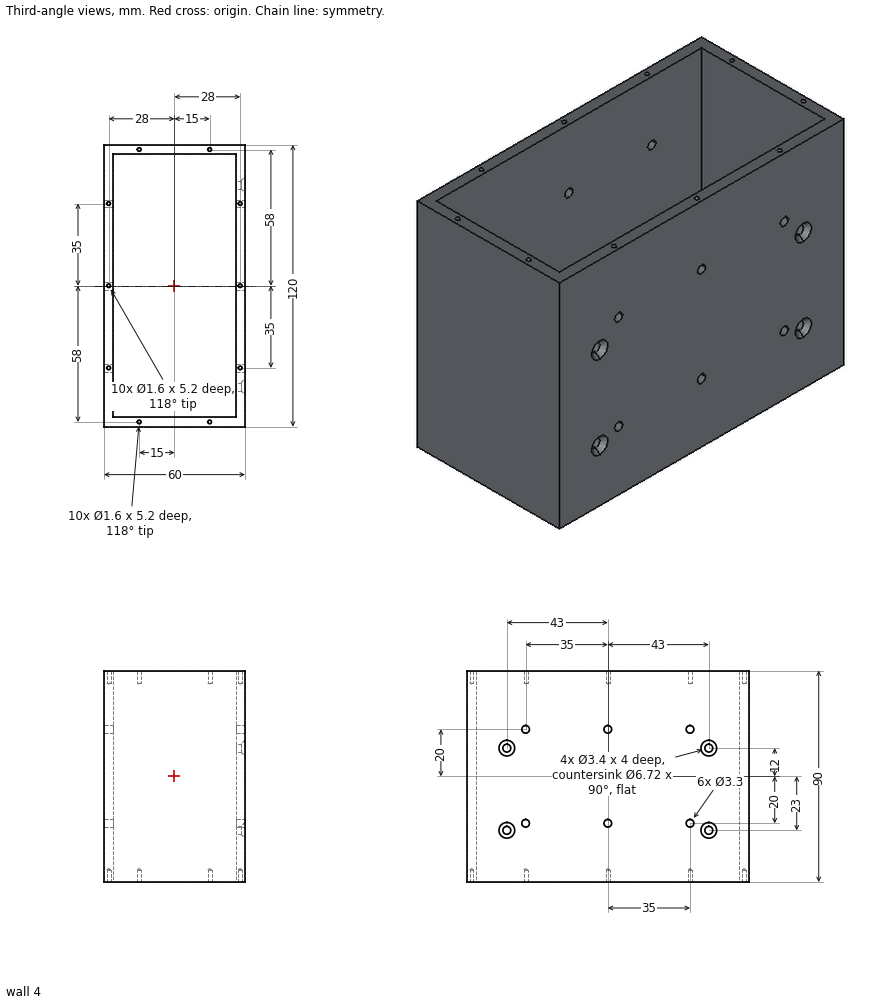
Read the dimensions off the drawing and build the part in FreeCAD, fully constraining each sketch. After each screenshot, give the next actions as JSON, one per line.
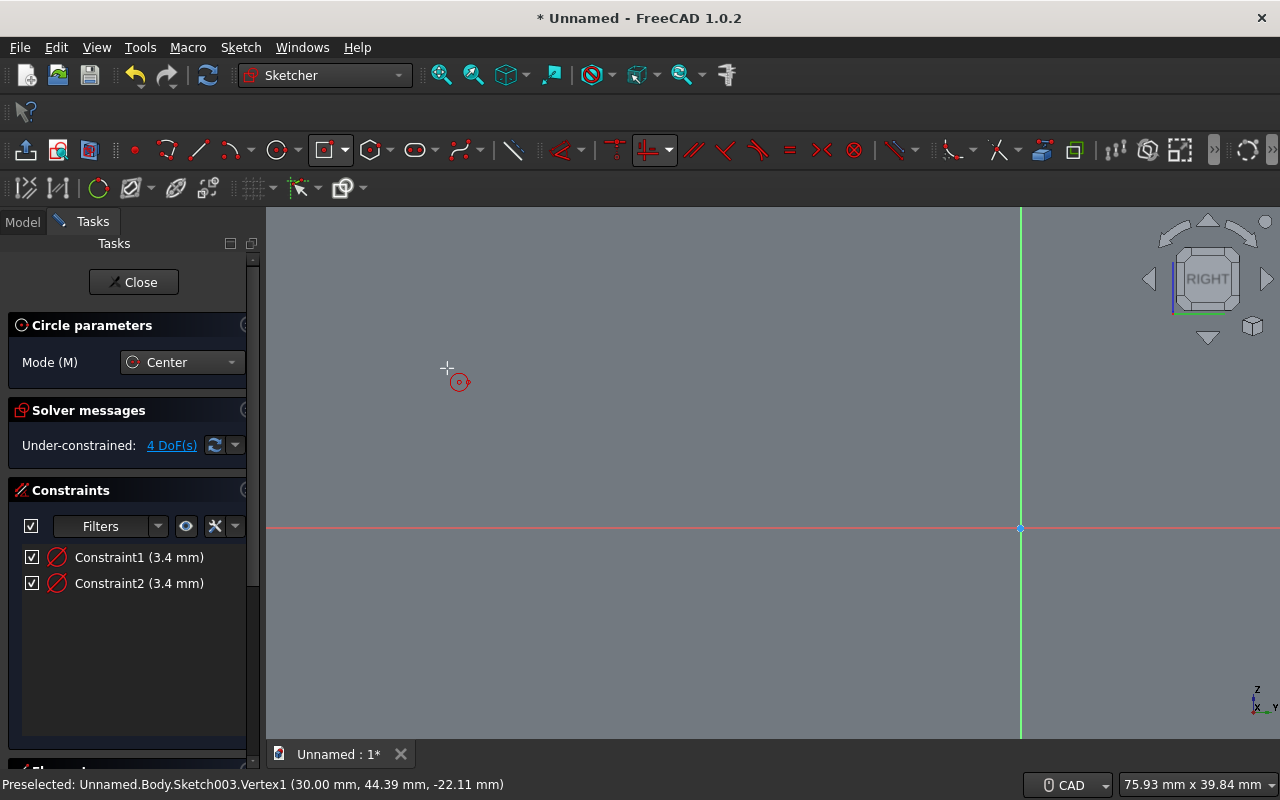
{"action": "left_click", "coordinate": [446, 368]}
{"action": "mouse_move", "coordinate": [462, 352]}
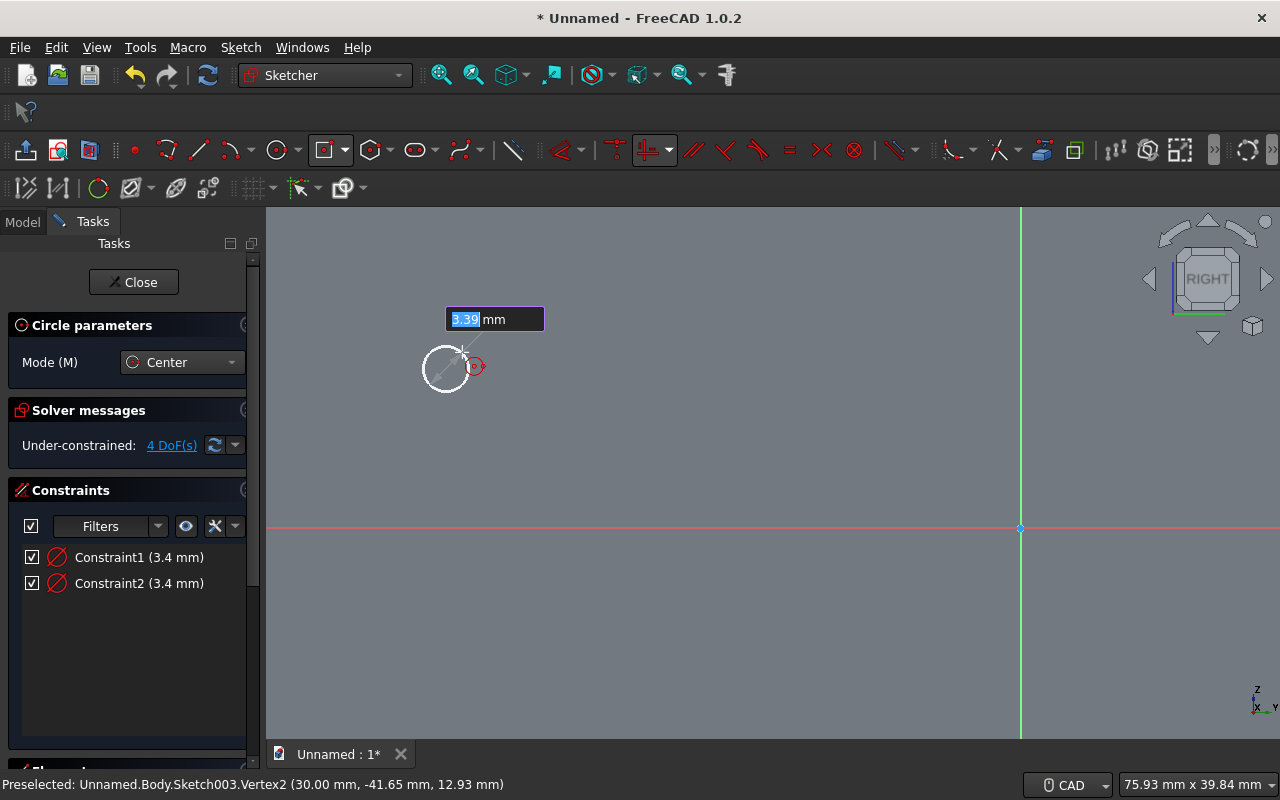
{"action": "type", "text": "3.4"}
{"action": "key", "text": "Return"}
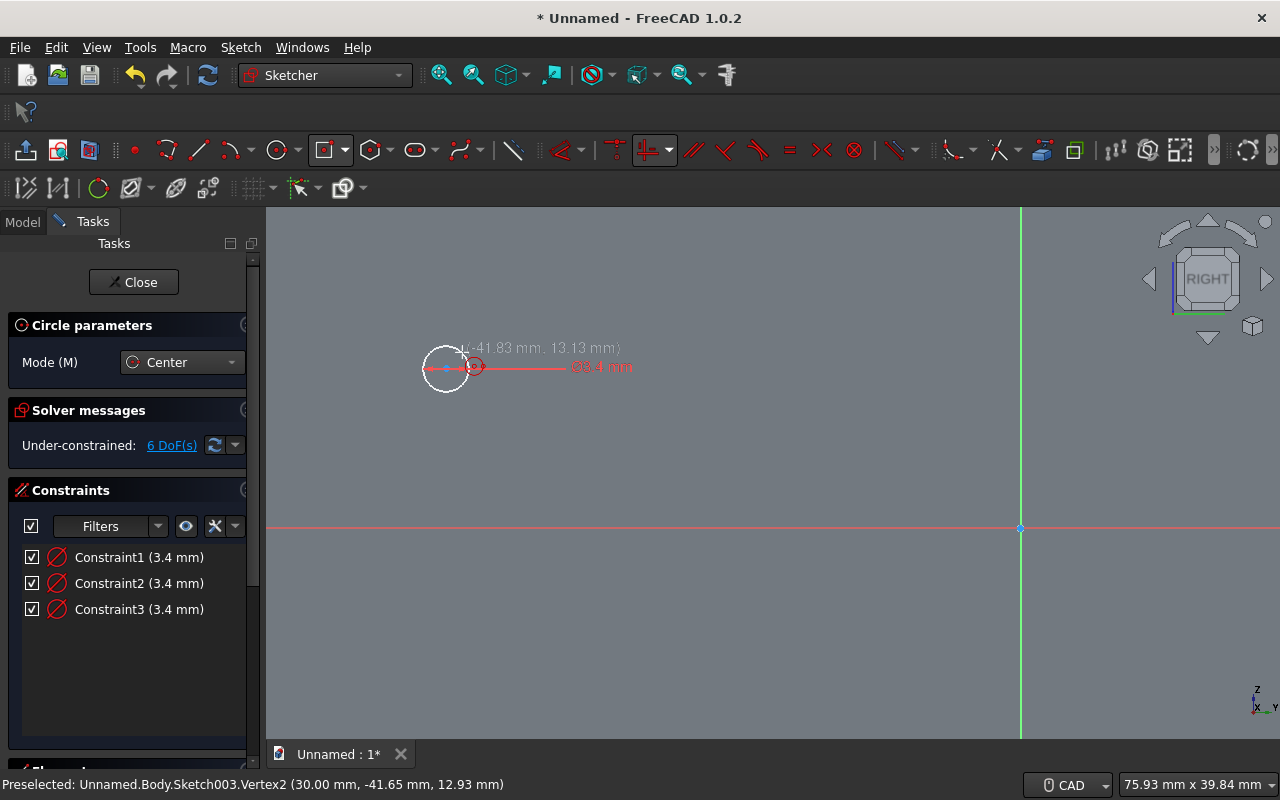
{"action": "scroll", "coordinate": [447, 368], "scroll_direction": "down", "scroll_amount": 4}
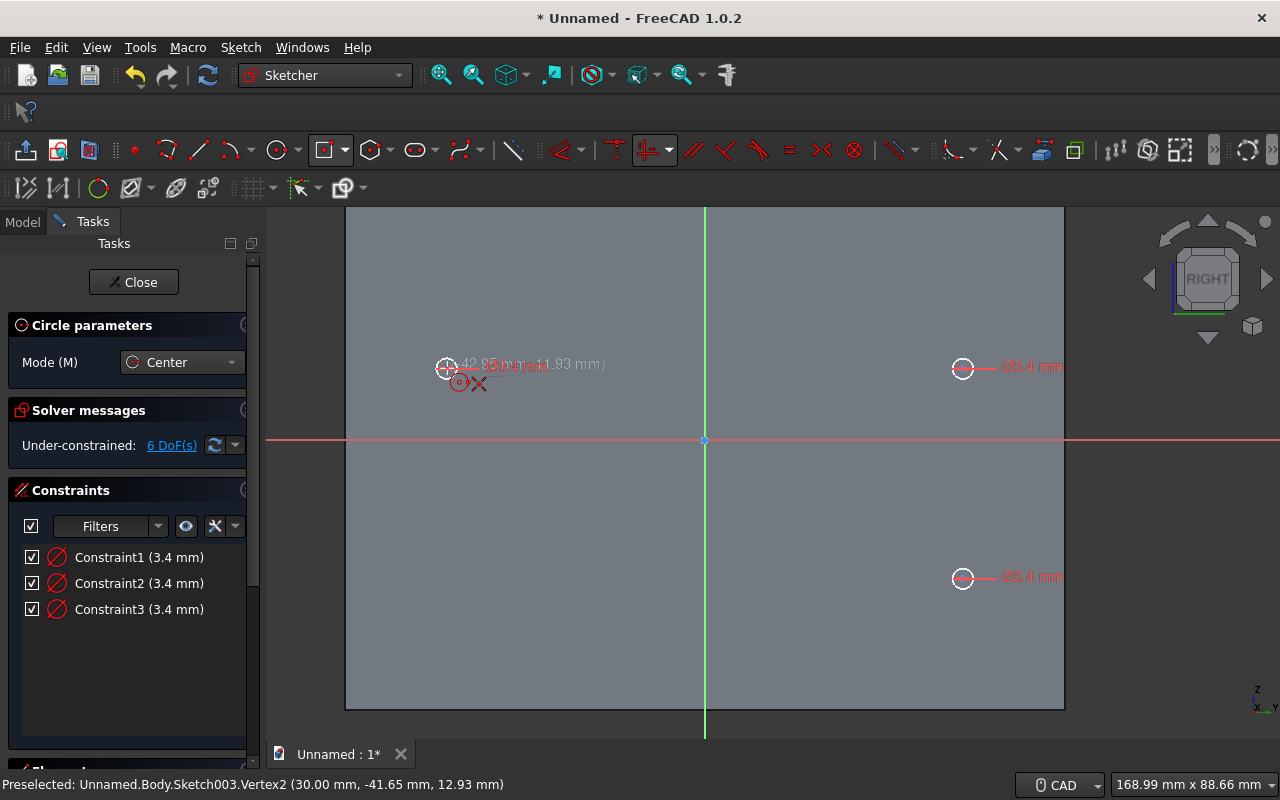
{"action": "scroll", "coordinate": [447, 578], "scroll_direction": "up", "scroll_amount": 4}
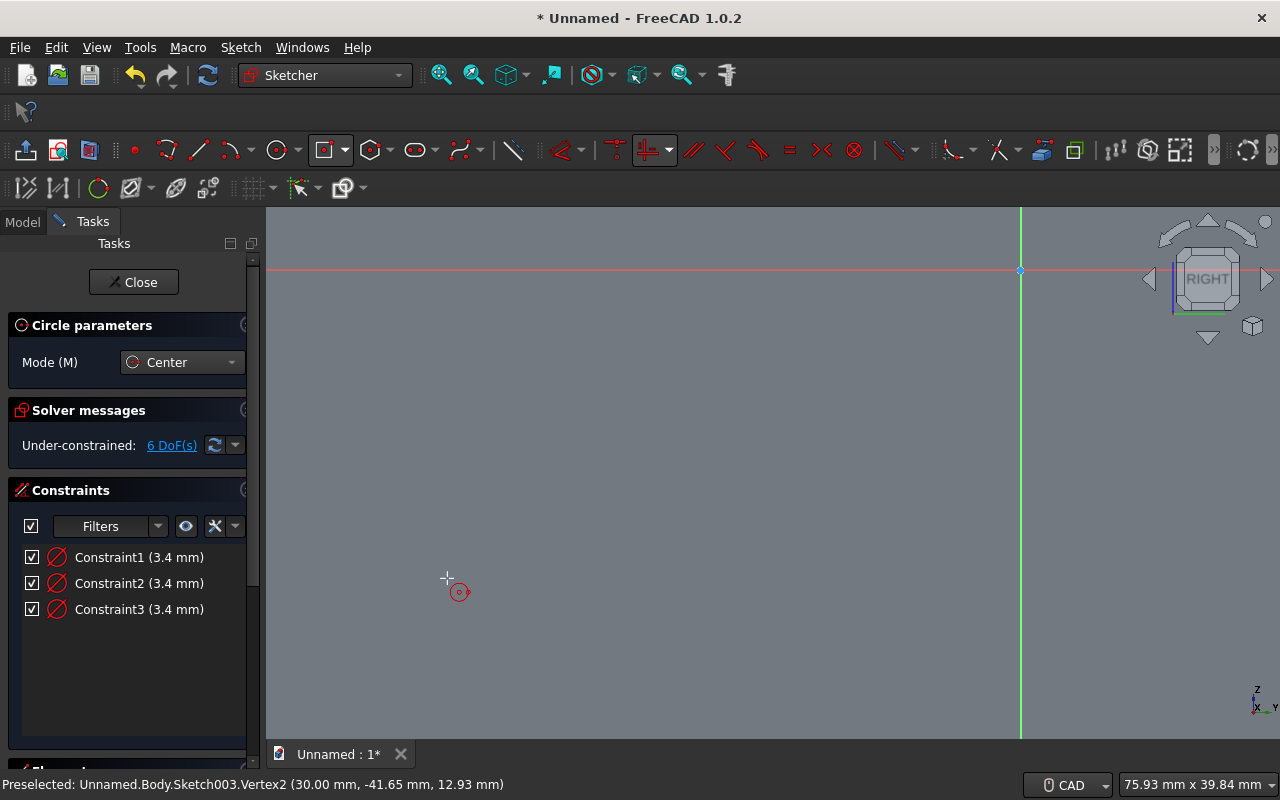
{"action": "left_click", "coordinate": [446, 578]}
{"action": "mouse_move", "coordinate": [462, 562]}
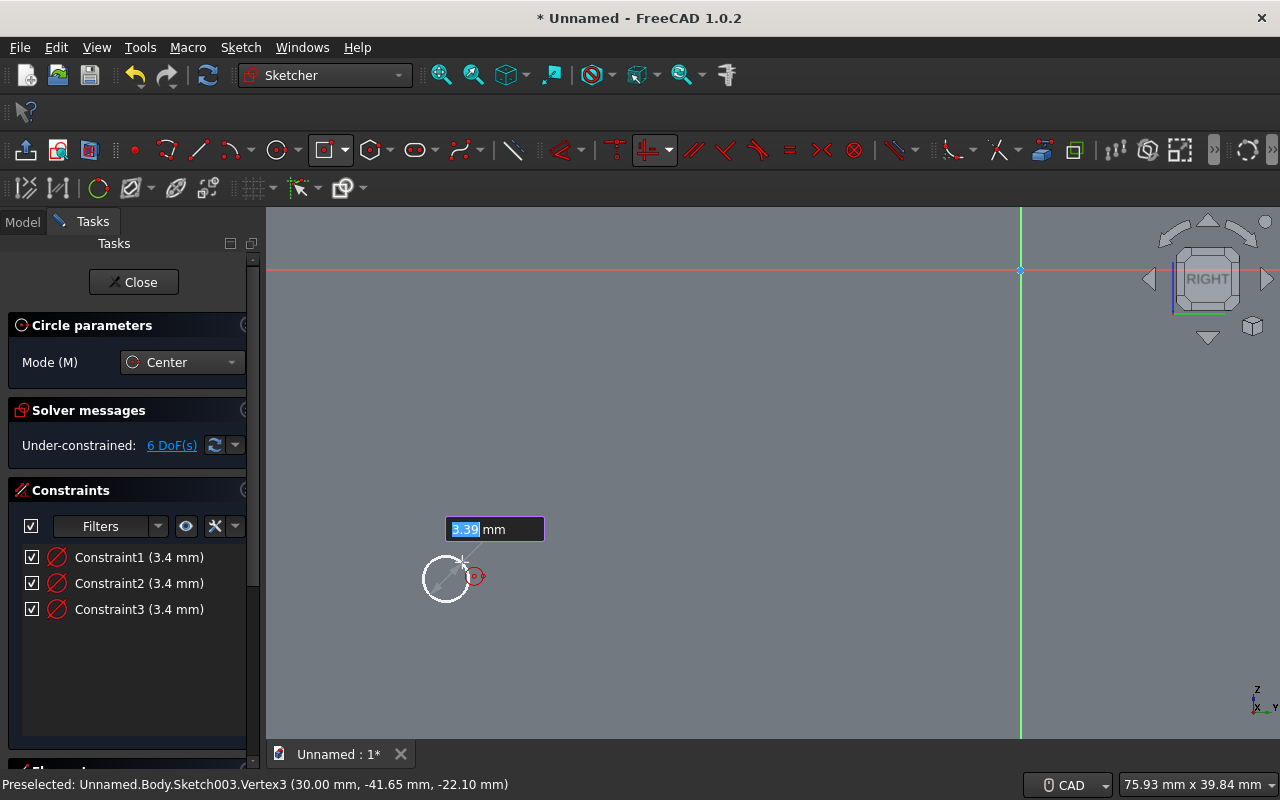
{"action": "type", "text": "3.4"}
{"action": "key", "text": "Return"}
{"action": "key", "text": "Escape"}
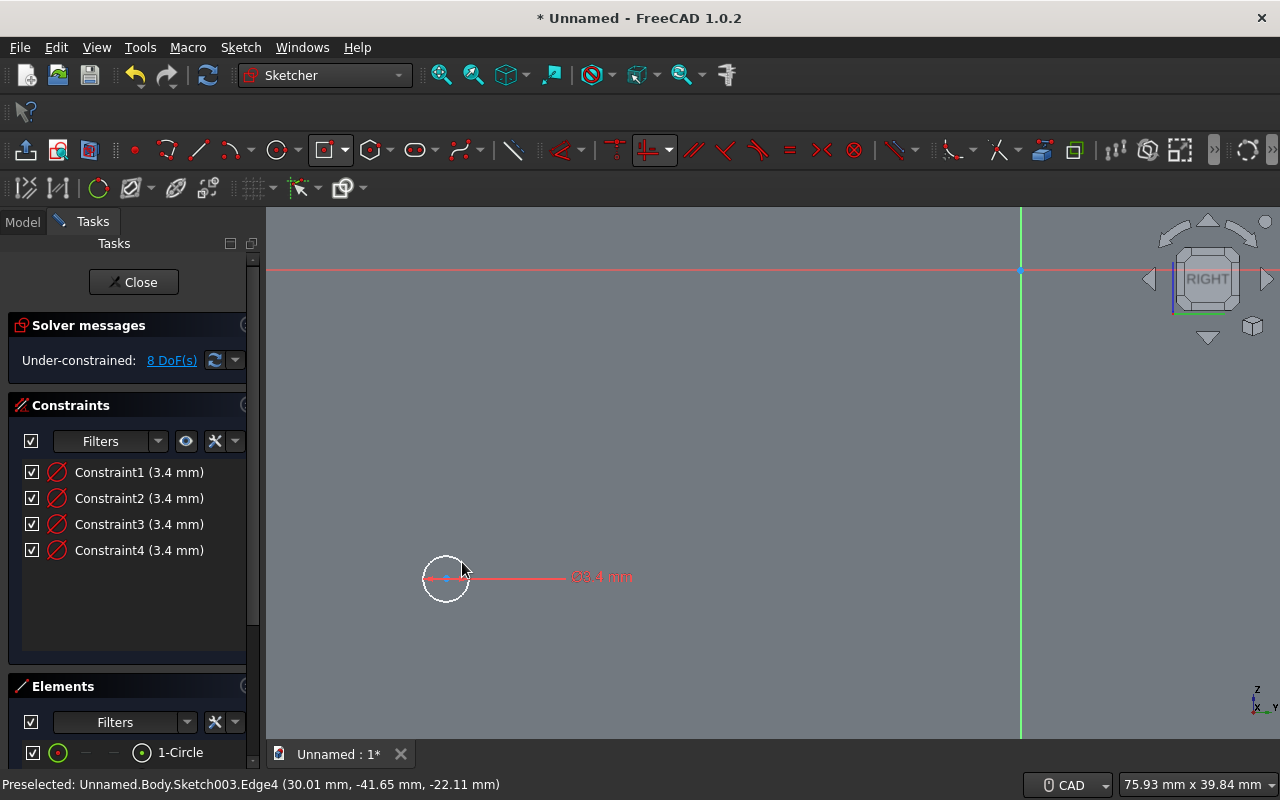
{"action": "scroll", "coordinate": [447, 578], "scroll_direction": "down", "scroll_amount": 4}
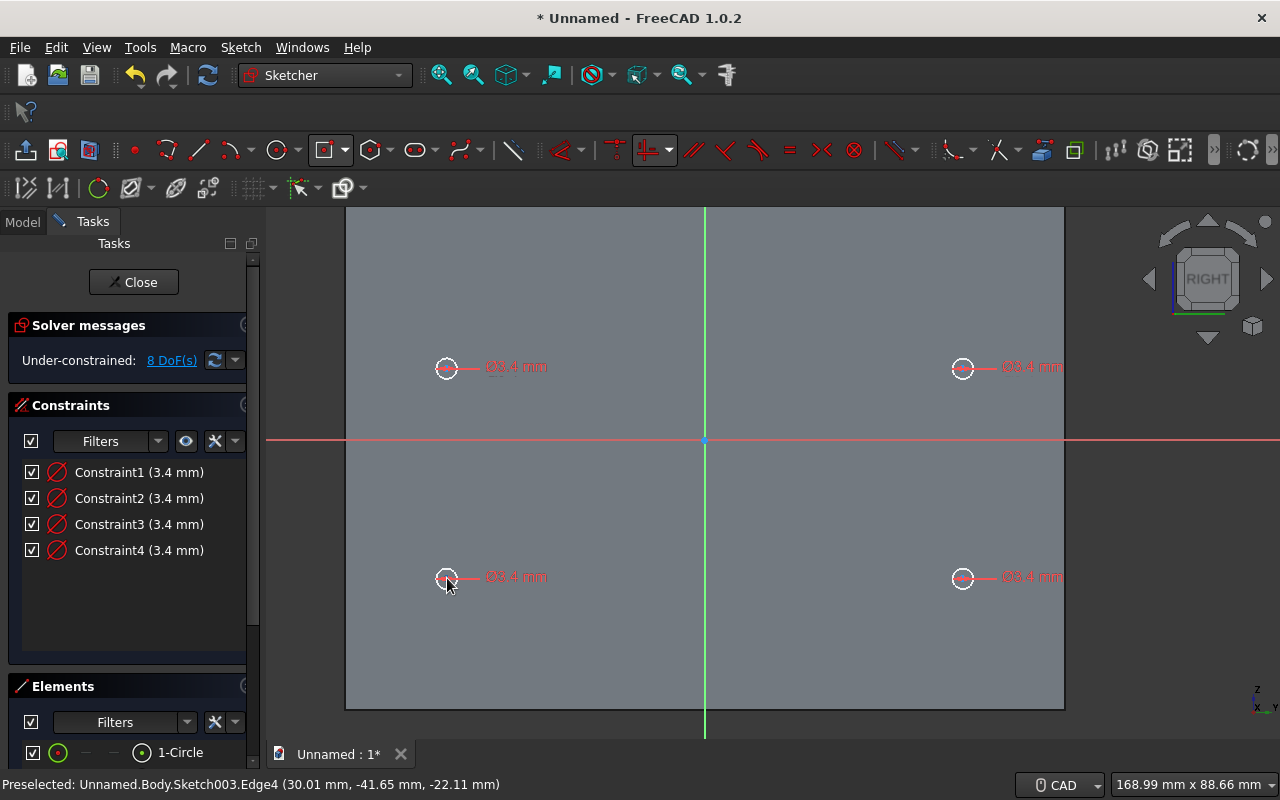
{"action": "left_click", "coordinate": [963, 369]}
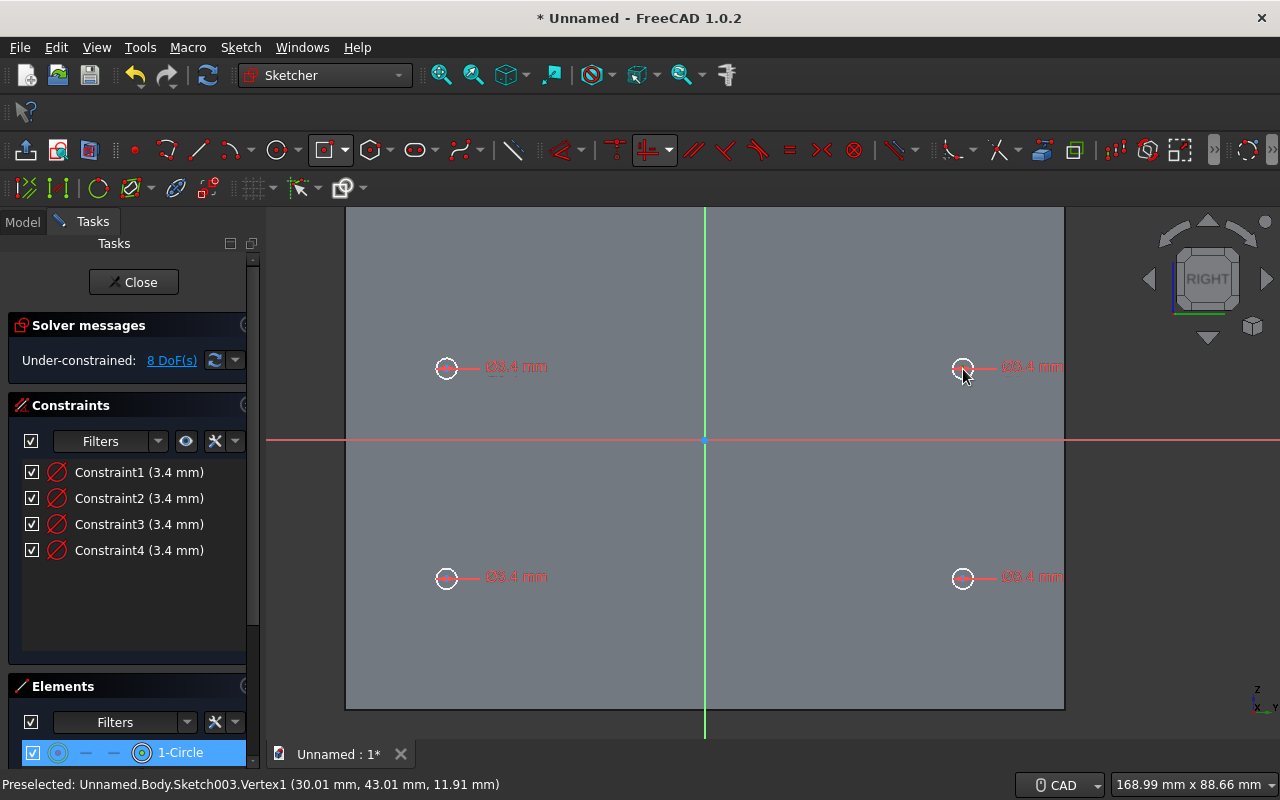
{"action": "left_click", "coordinate": [963, 579]}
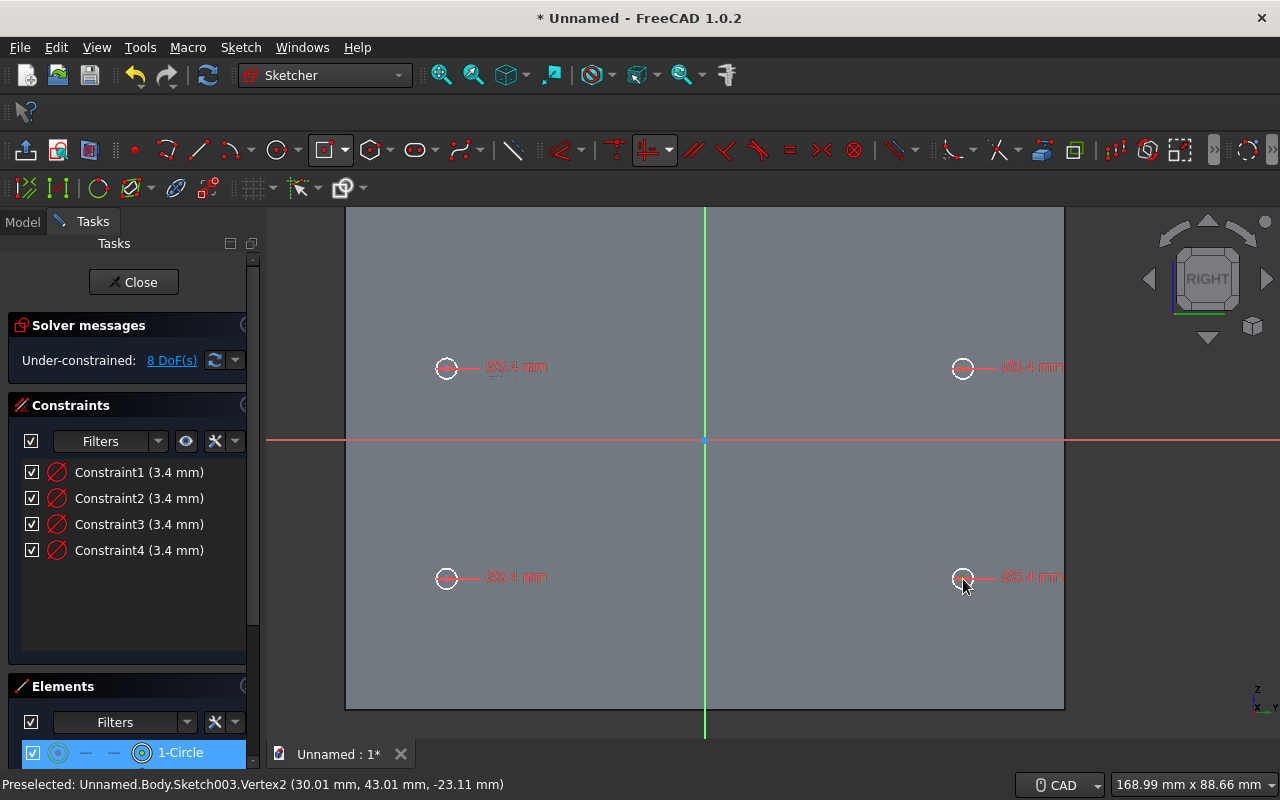
{"action": "left_click", "coordinate": [672, 150]}